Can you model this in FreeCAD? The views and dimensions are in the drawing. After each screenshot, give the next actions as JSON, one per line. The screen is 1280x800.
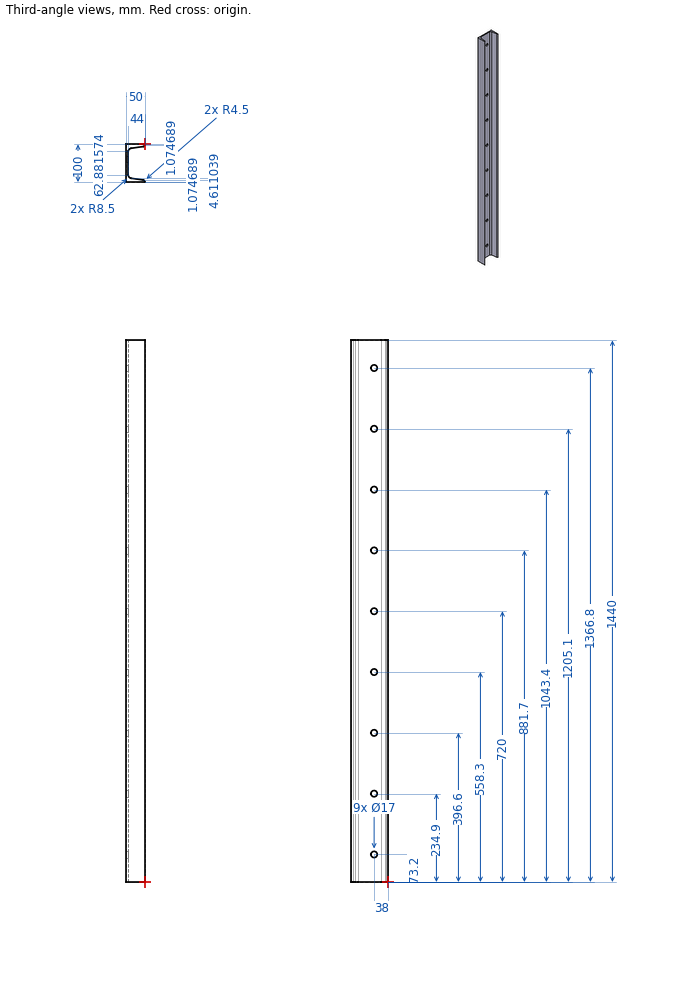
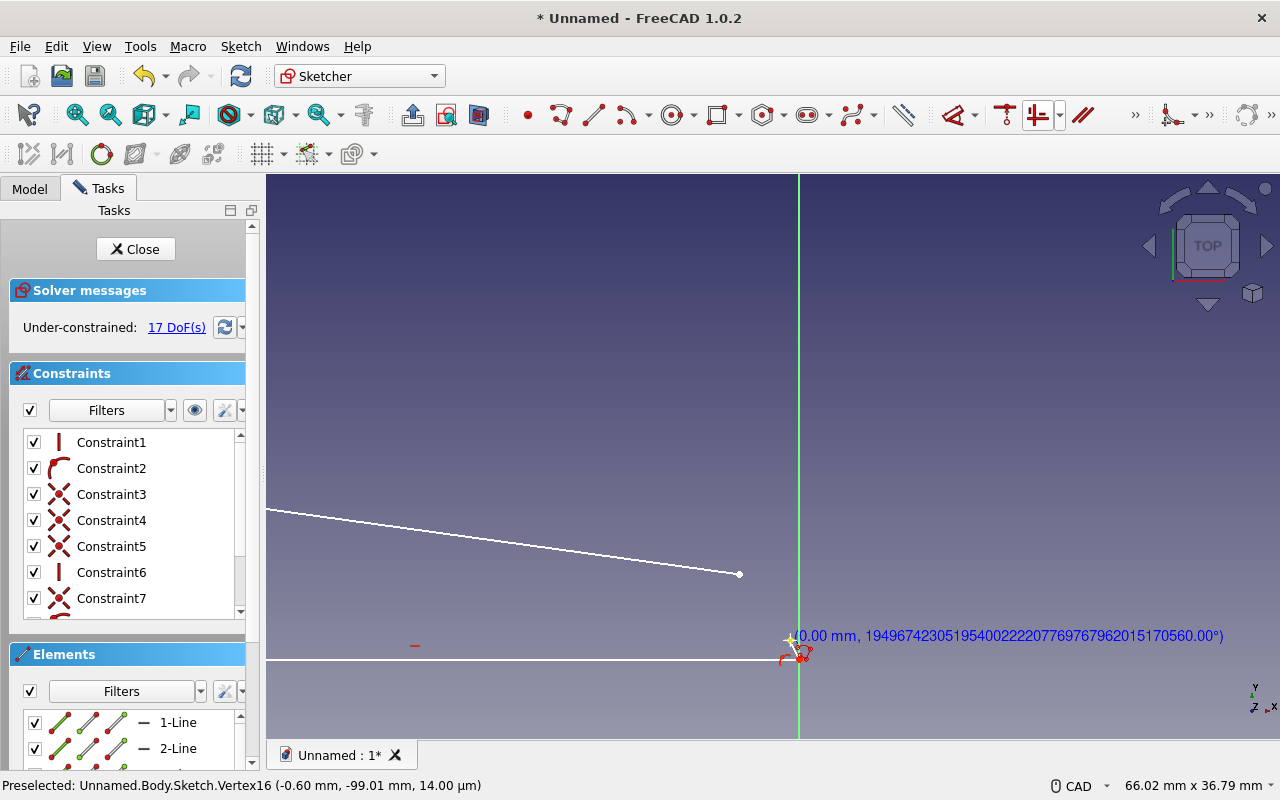
{"action": "key", "text": "g 3 a"}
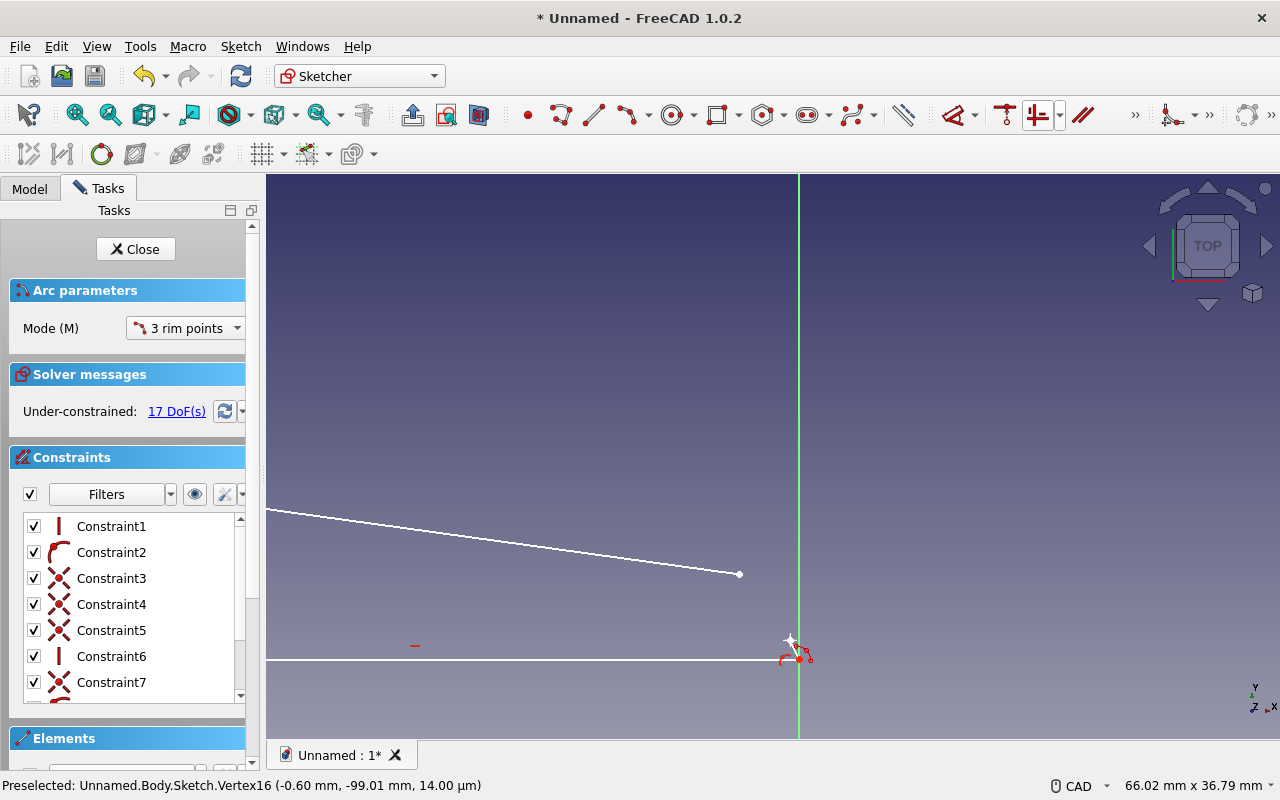
{"action": "scroll", "coordinate": [799, 643], "scroll_direction": "down", "scroll_amount": 7}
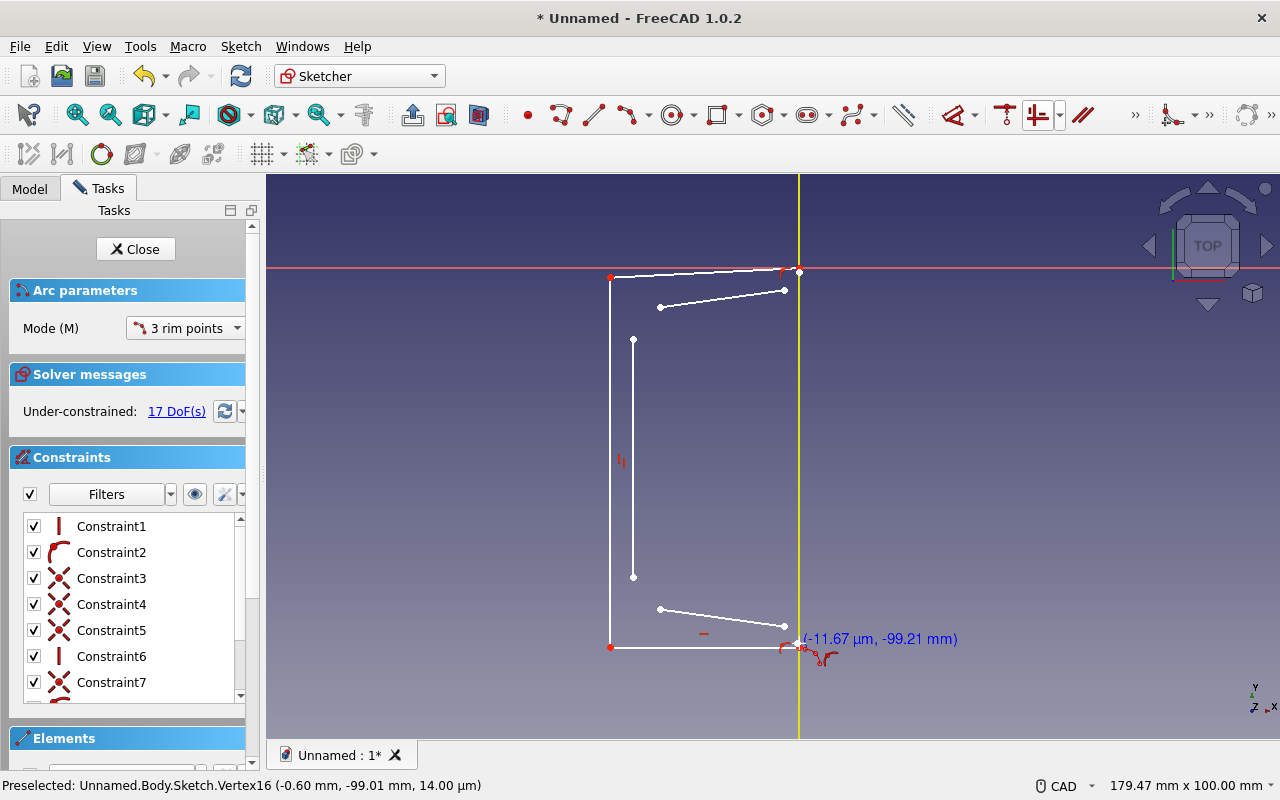
{"action": "left_click", "coordinate": [660, 610]}
{"action": "left_click", "coordinate": [633, 578]}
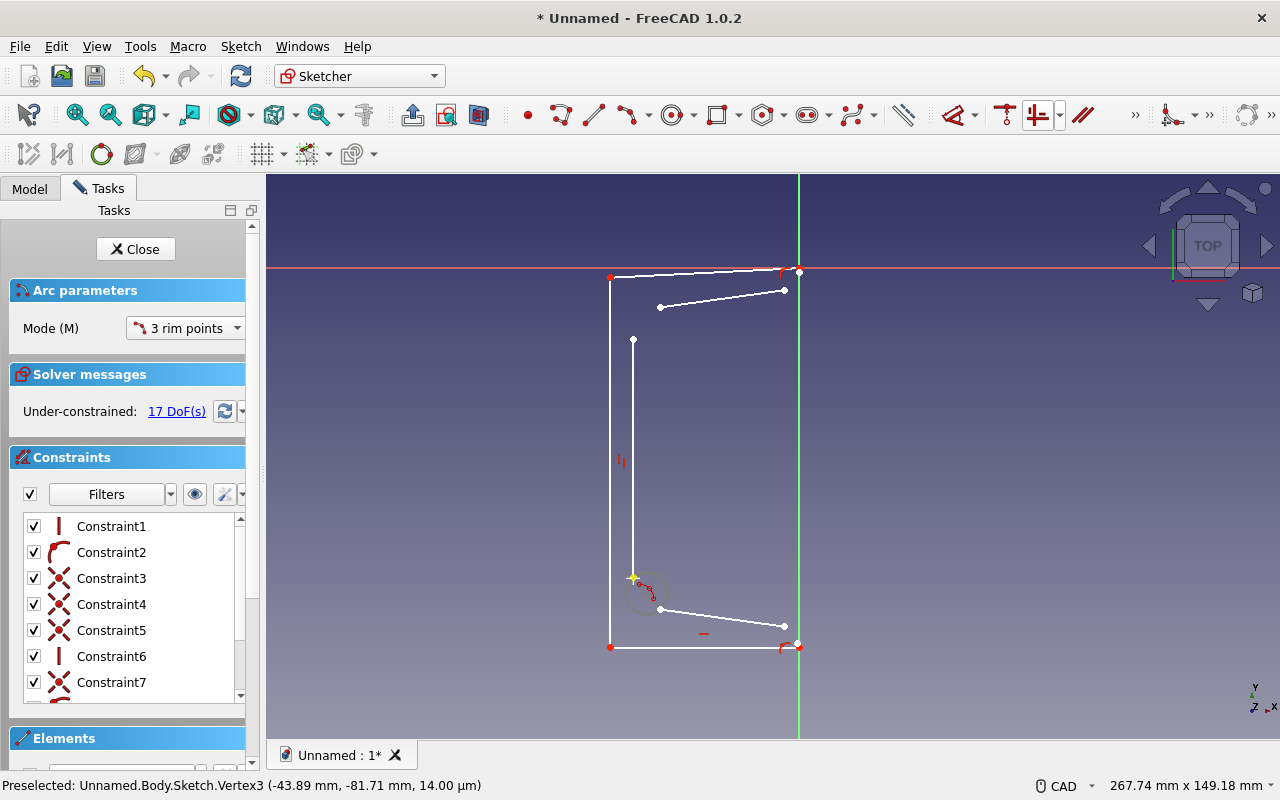
{"action": "scroll", "coordinate": [641, 598], "scroll_direction": "up", "scroll_amount": 4}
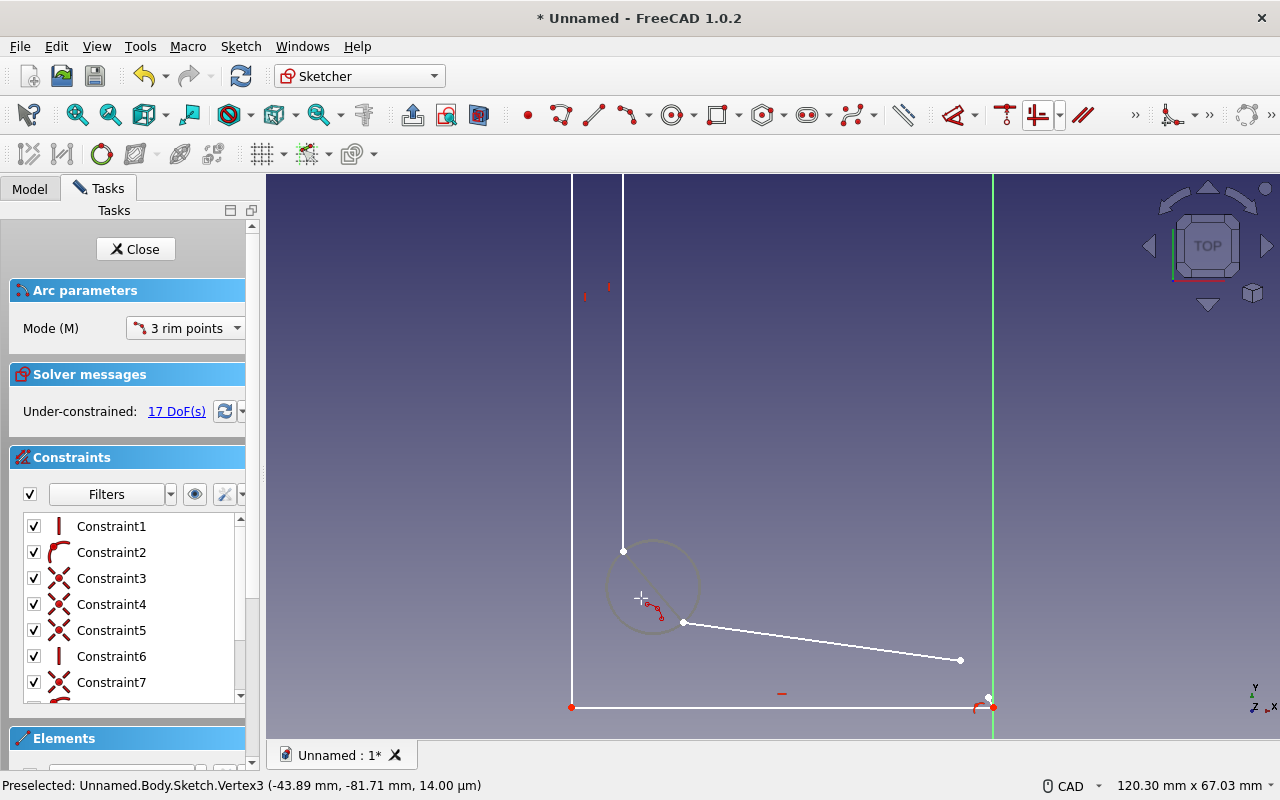
{"action": "left_click", "coordinate": [640, 596]}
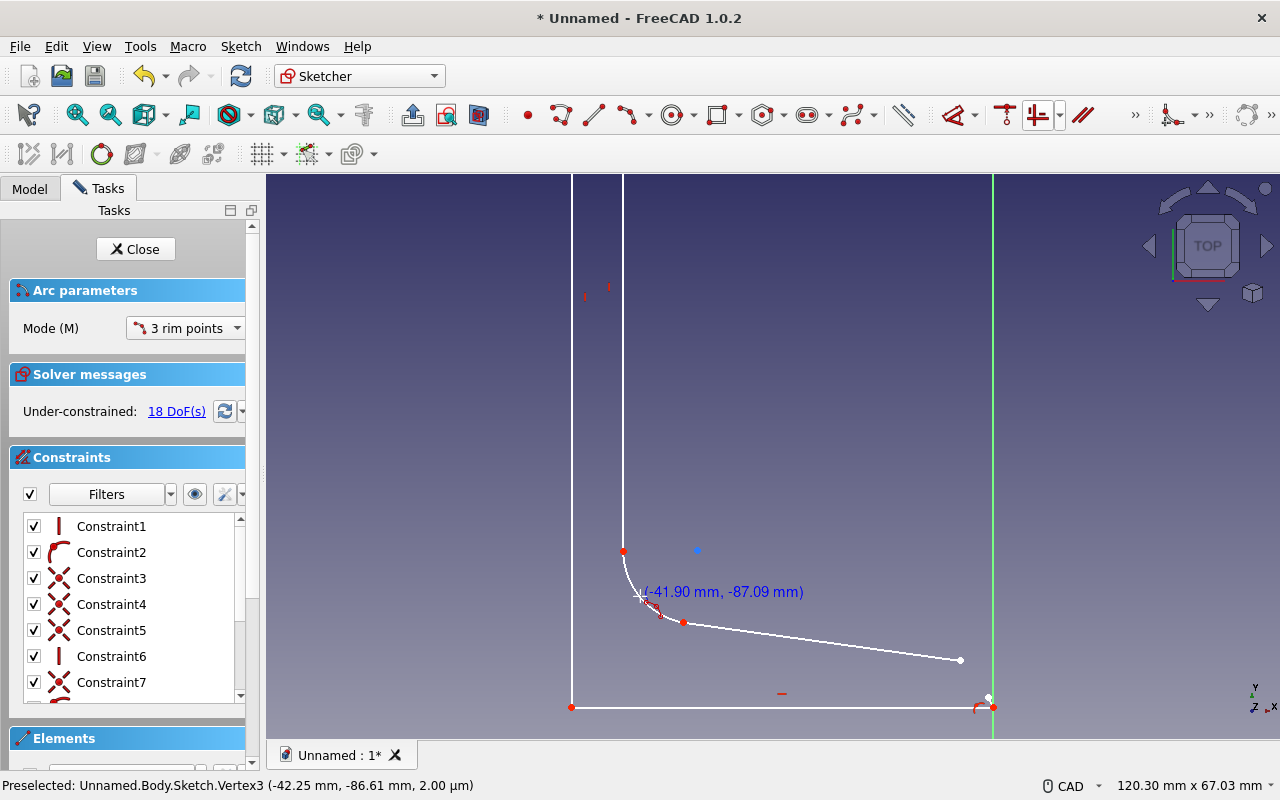
{"action": "scroll", "coordinate": [641, 597], "scroll_direction": "down", "scroll_amount": 4}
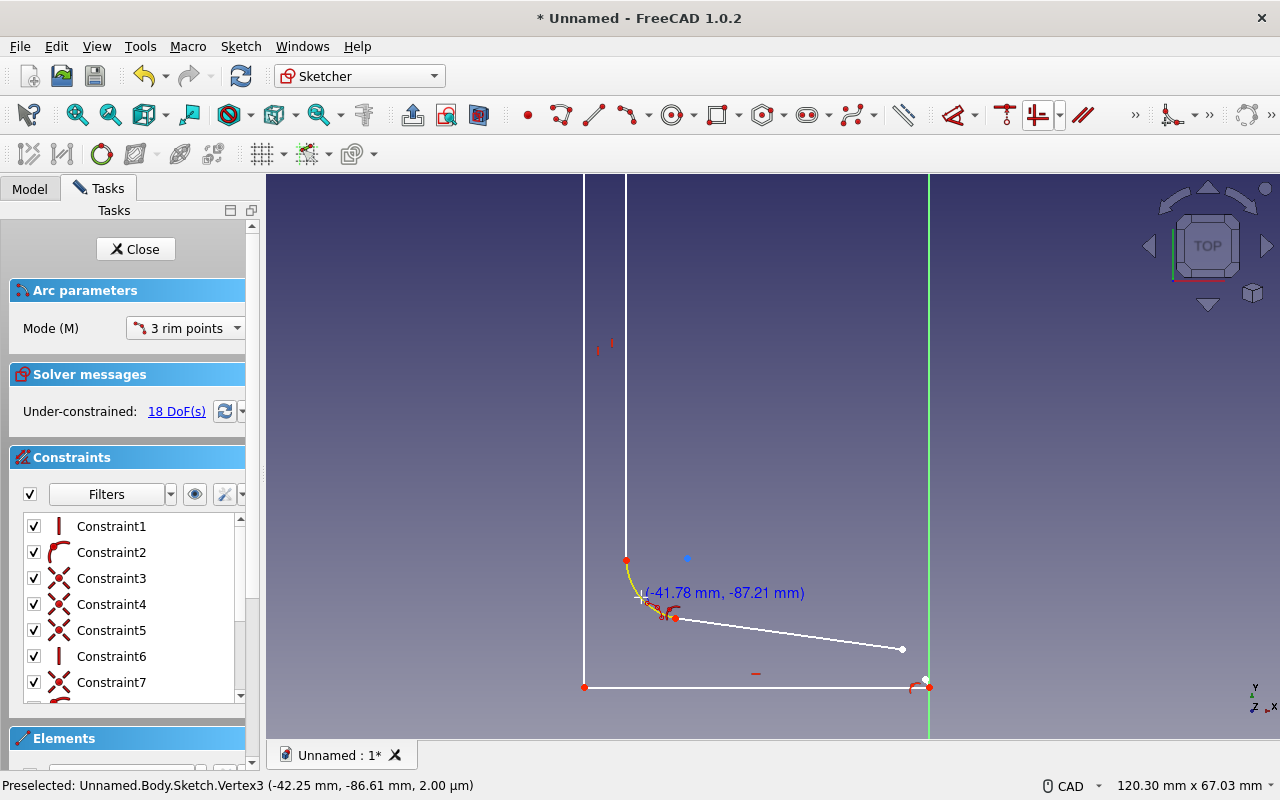
{"action": "left_click", "coordinate": [633, 339]}
{"action": "left_click", "coordinate": [660, 307]}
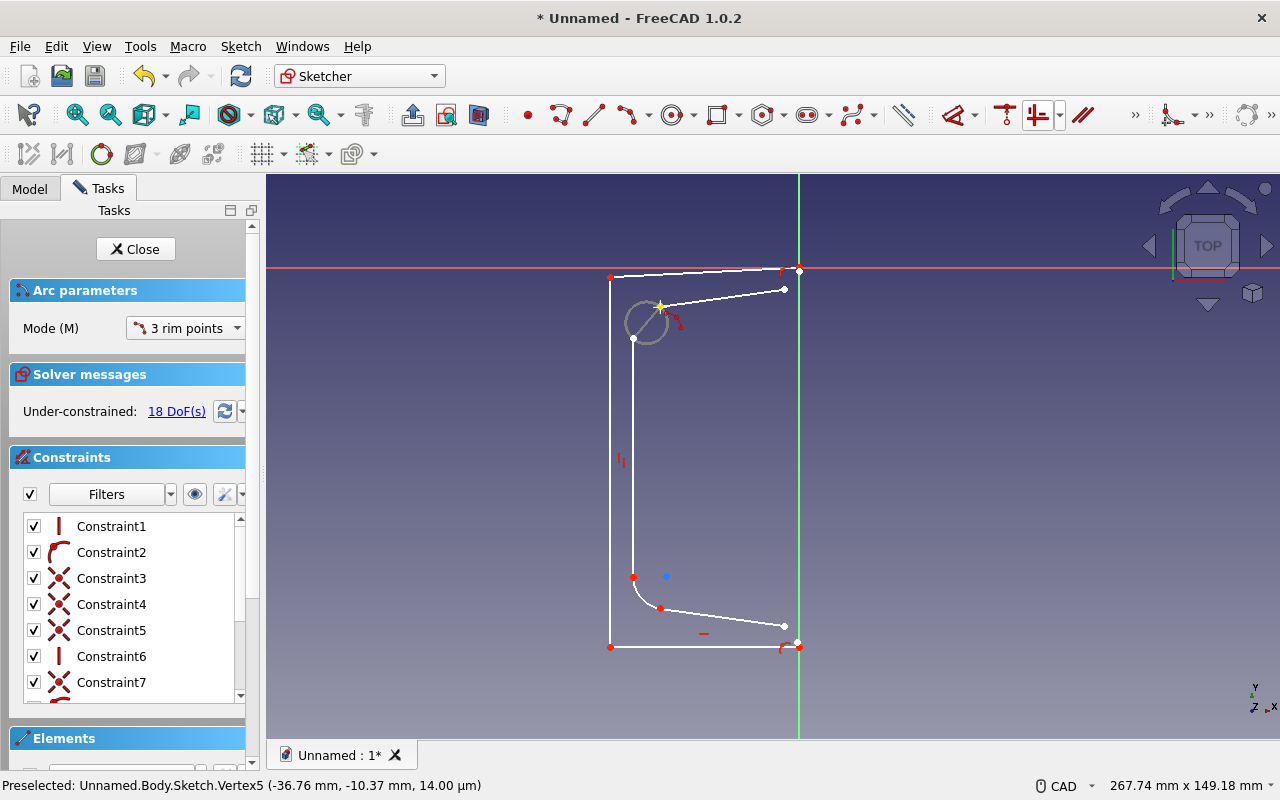
{"action": "scroll", "coordinate": [641, 317], "scroll_direction": "up", "scroll_amount": 4}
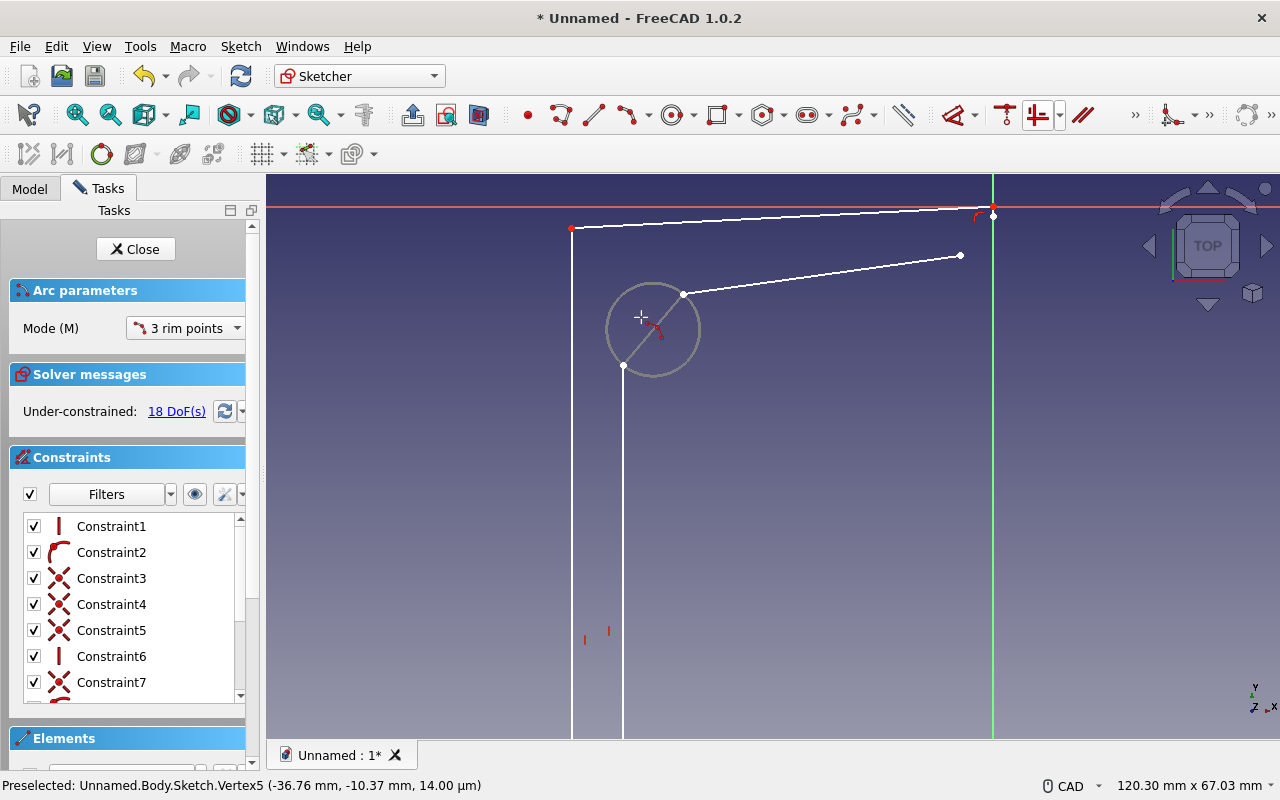
{"action": "left_click", "coordinate": [640, 316]}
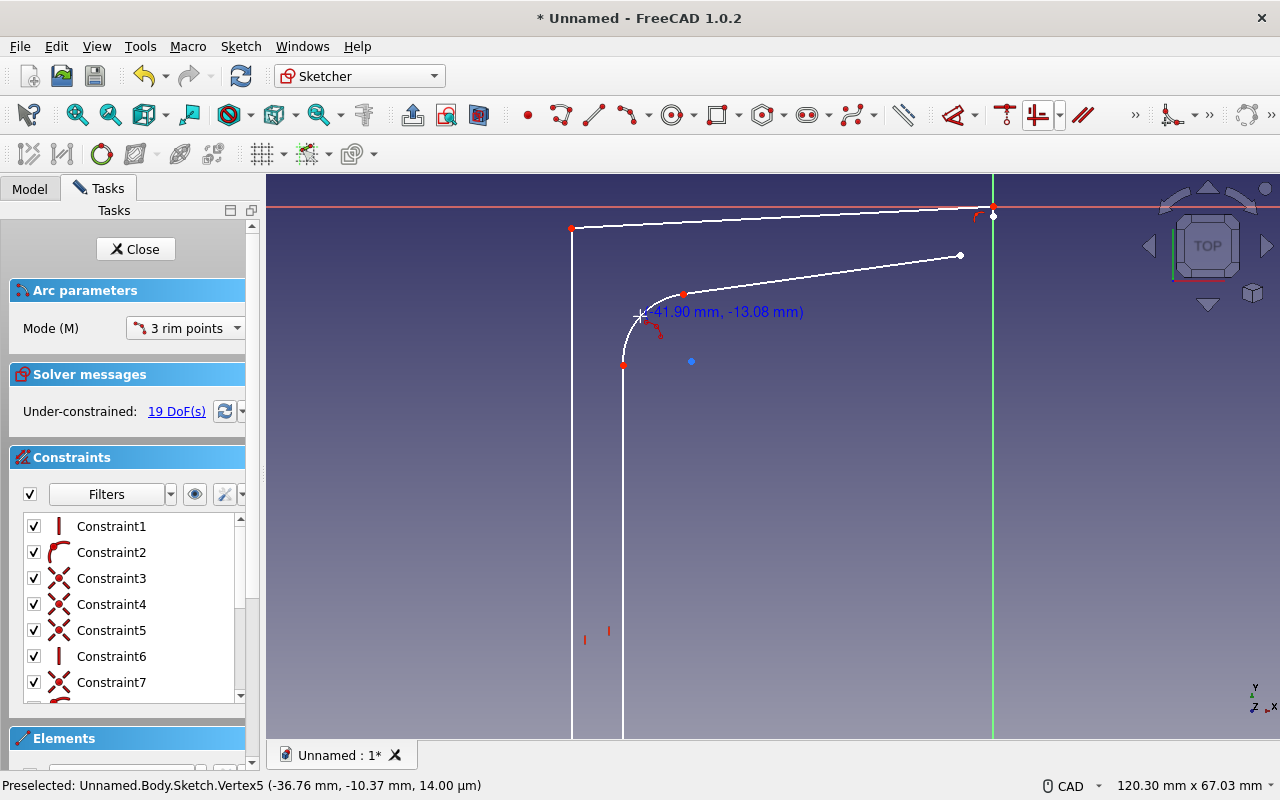
{"action": "left_click", "coordinate": [960, 256]}